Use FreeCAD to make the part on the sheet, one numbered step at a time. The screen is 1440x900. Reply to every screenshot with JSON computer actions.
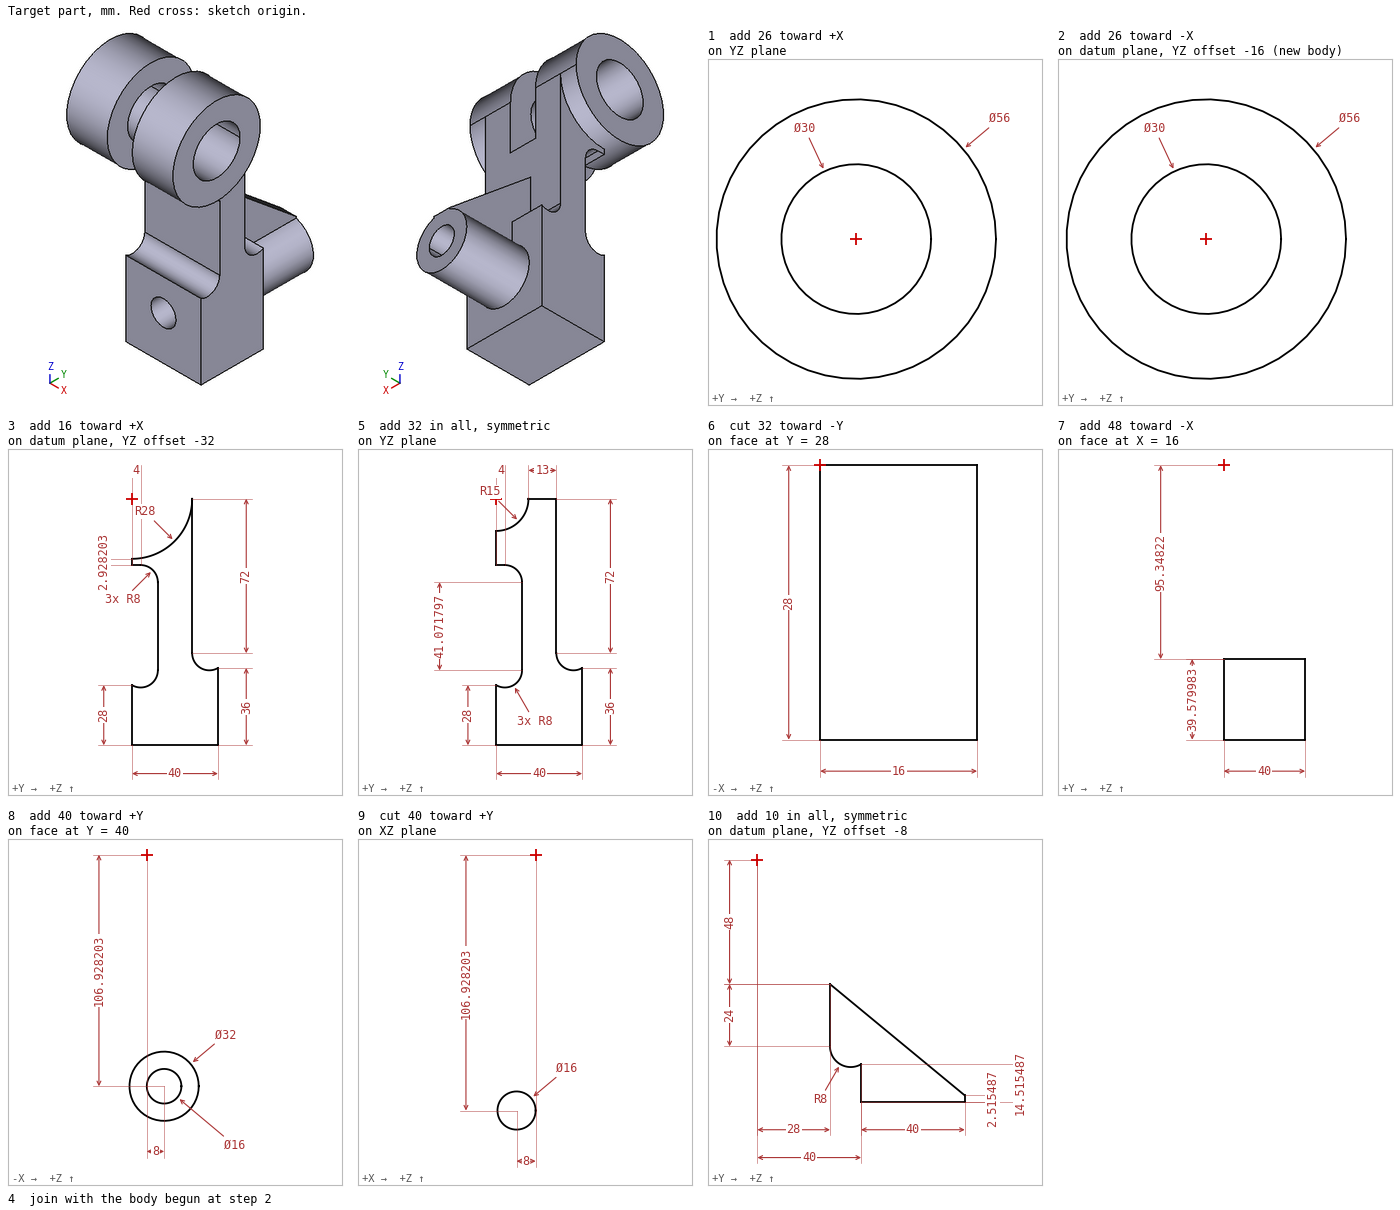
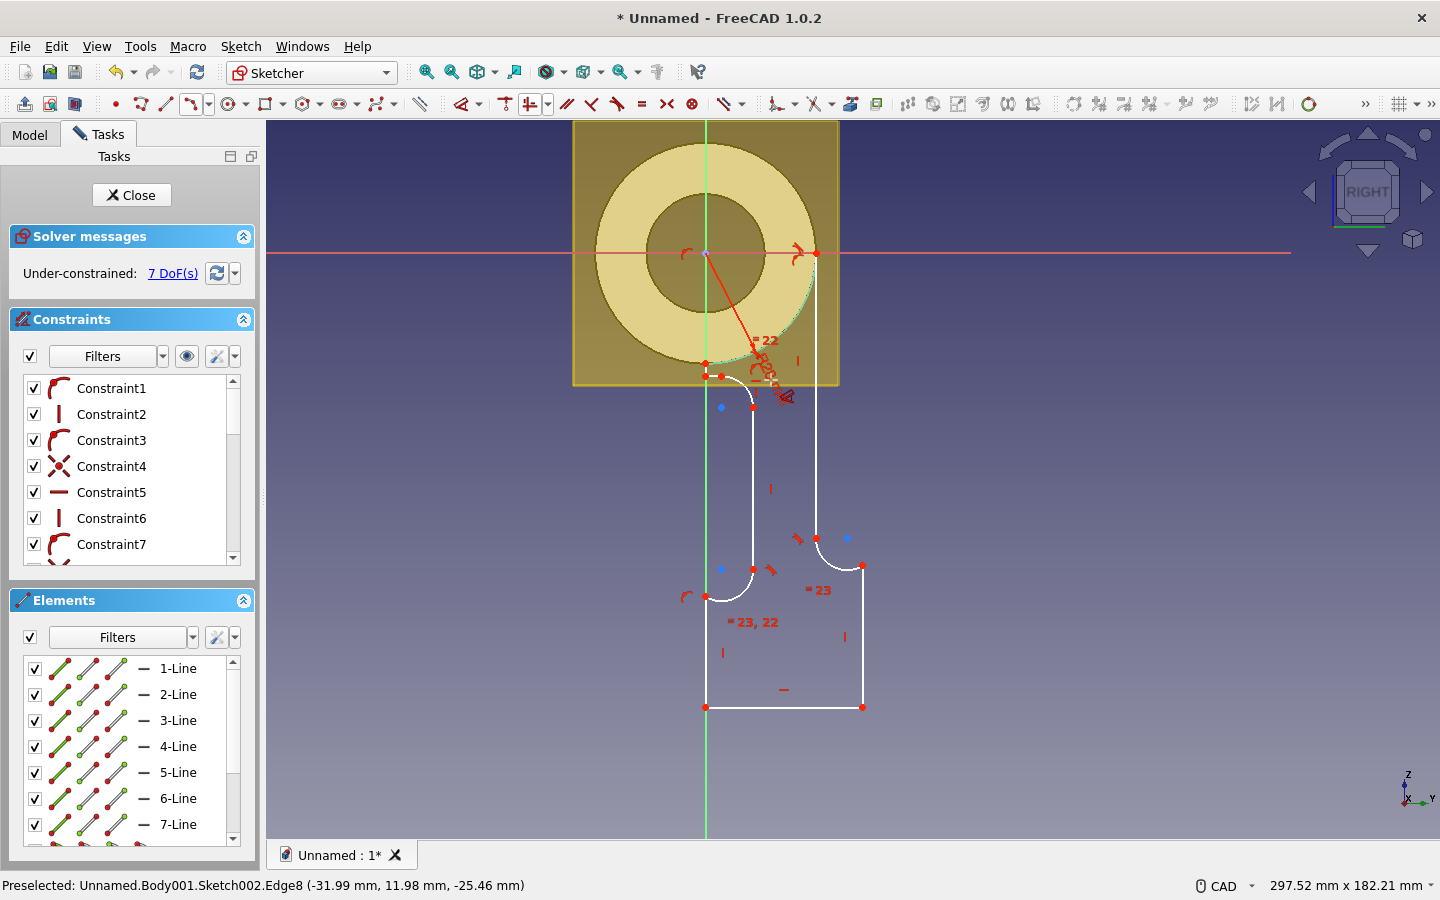
{"action": "scroll", "coordinate": [750, 393], "scroll_direction": "up", "scroll_amount": 2}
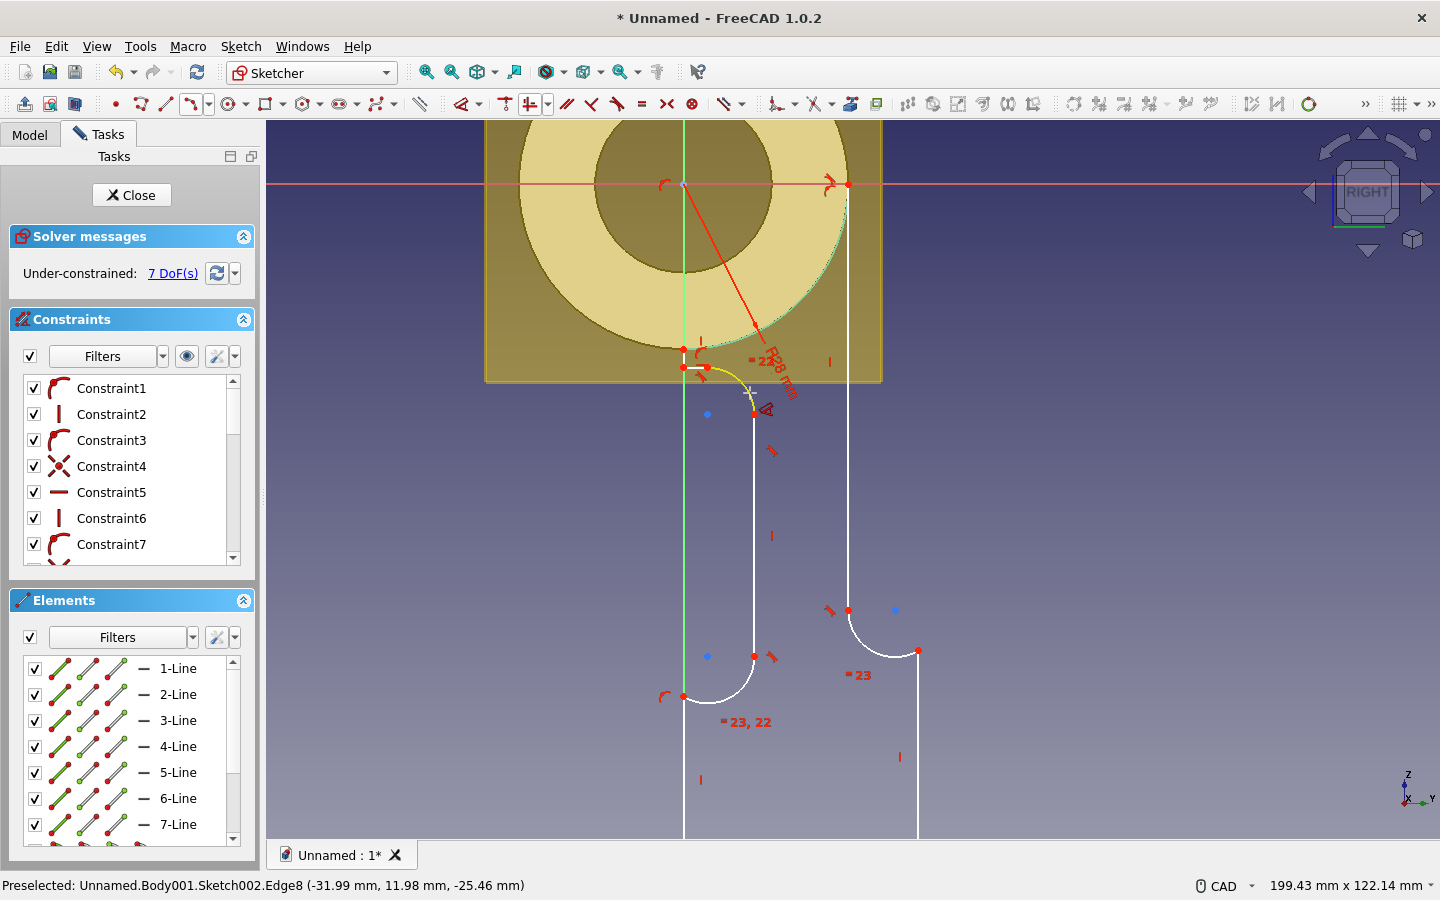
{"action": "left_click", "coordinate": [749, 393]}
{"action": "left_click", "coordinate": [786, 416]}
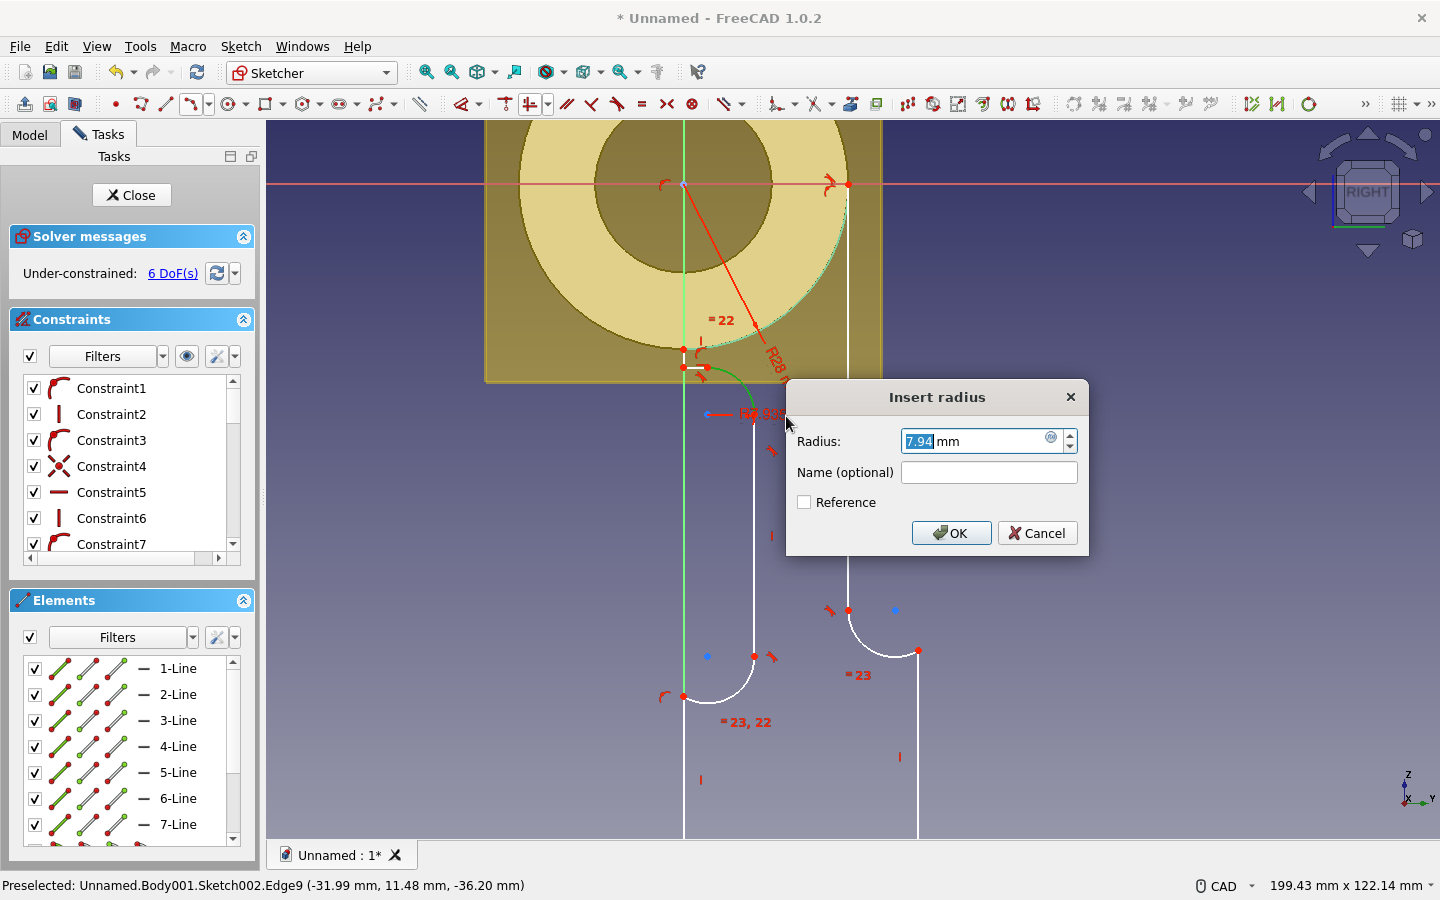
{"action": "type", "text": "8"}
{"action": "key", "text": "Return"}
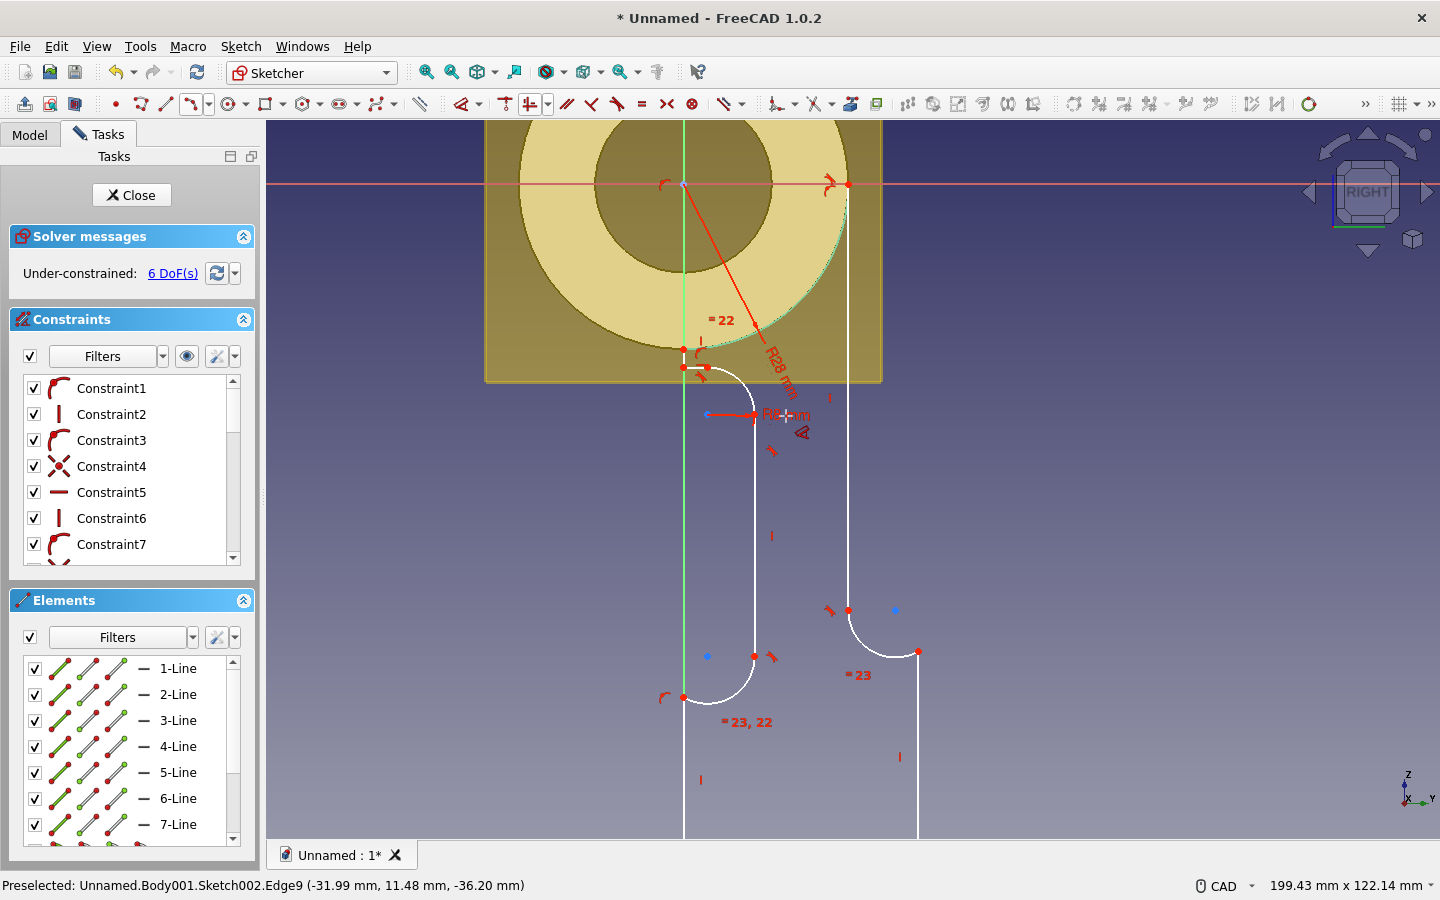
{"action": "scroll", "coordinate": [693, 368], "scroll_direction": "up", "scroll_amount": 3}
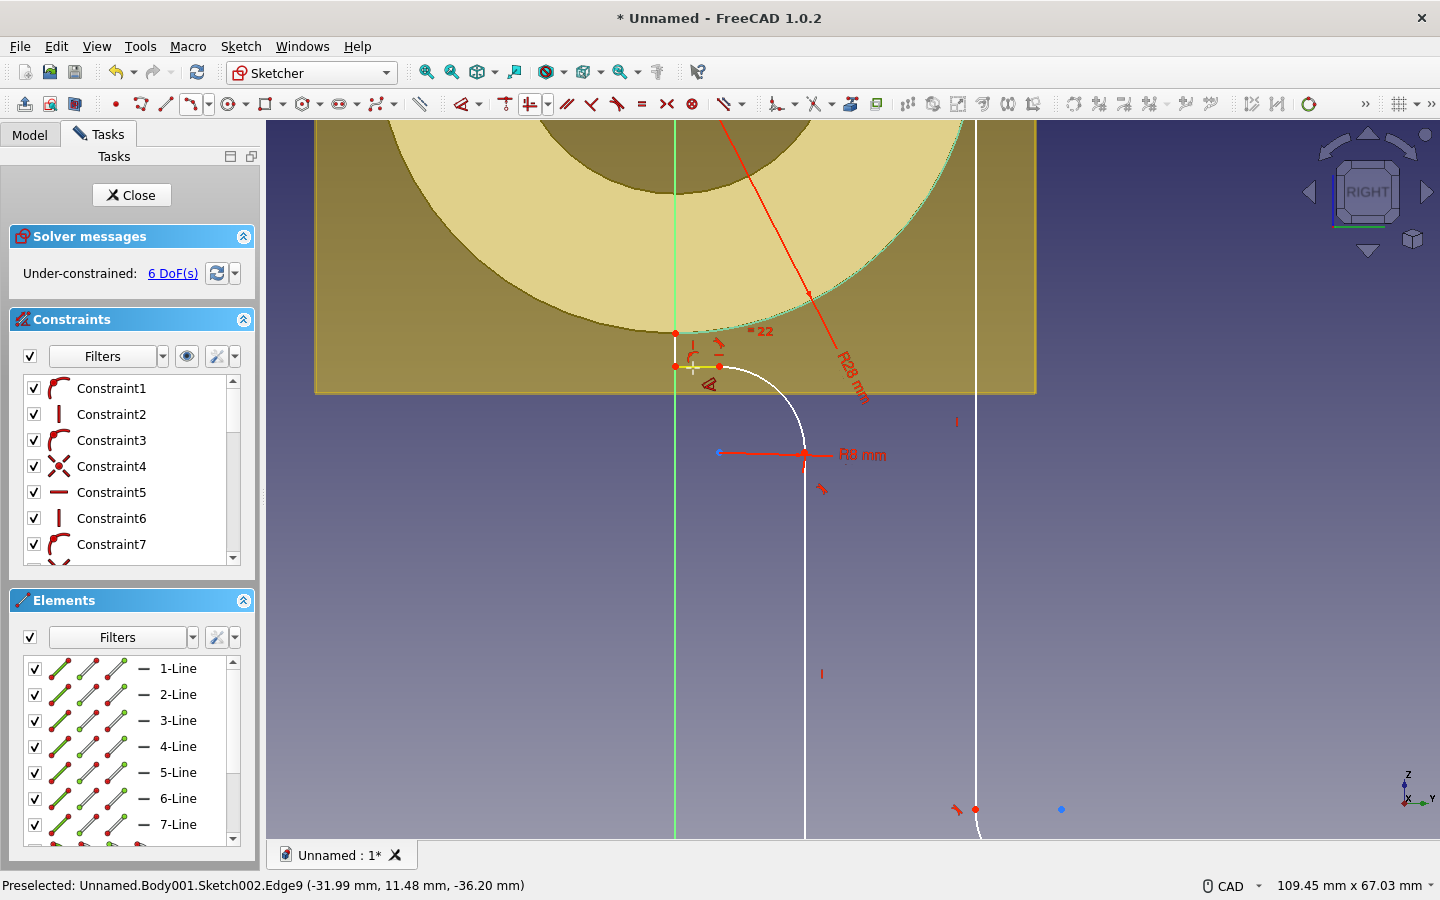
{"action": "left_click", "coordinate": [693, 367]}
{"action": "left_click", "coordinate": [697, 401]}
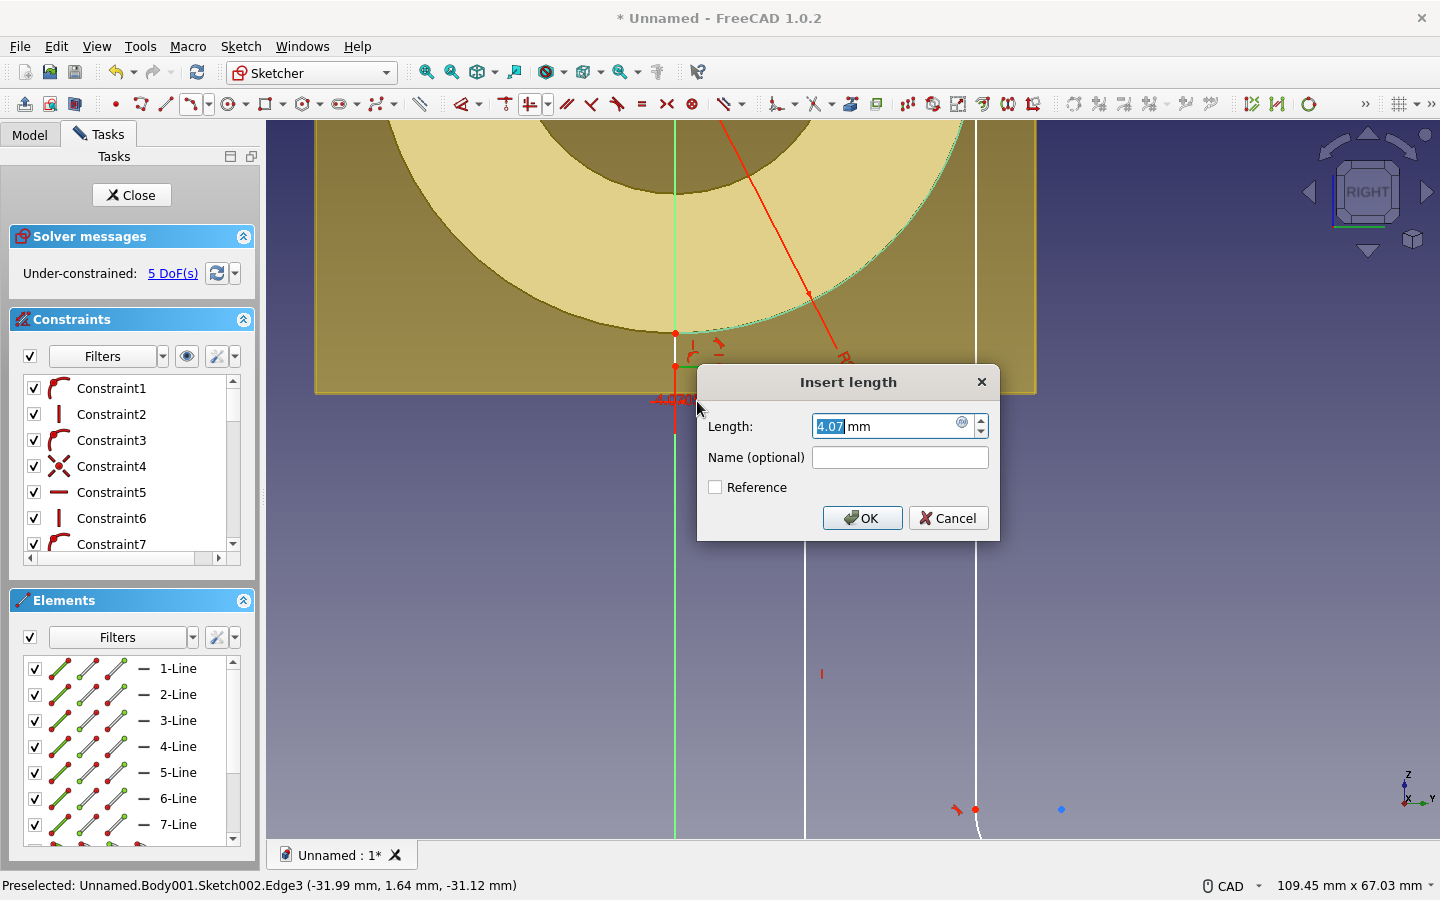
{"action": "type", "text": "4"}
{"action": "key", "text": "Return"}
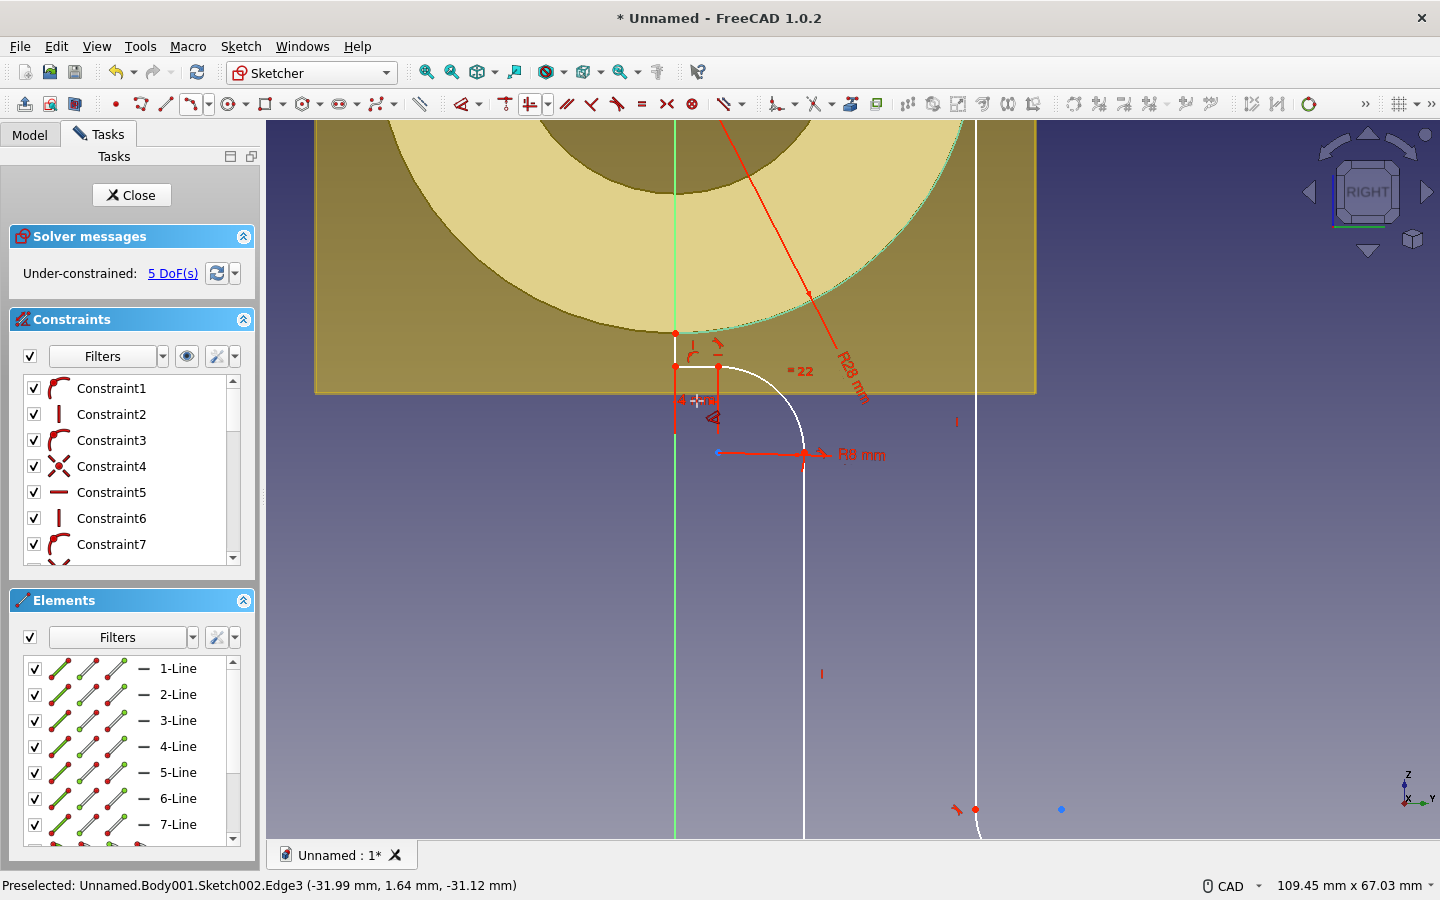
{"action": "left_click", "coordinate": [976, 576]}
{"action": "left_click", "coordinate": [1010, 479]}